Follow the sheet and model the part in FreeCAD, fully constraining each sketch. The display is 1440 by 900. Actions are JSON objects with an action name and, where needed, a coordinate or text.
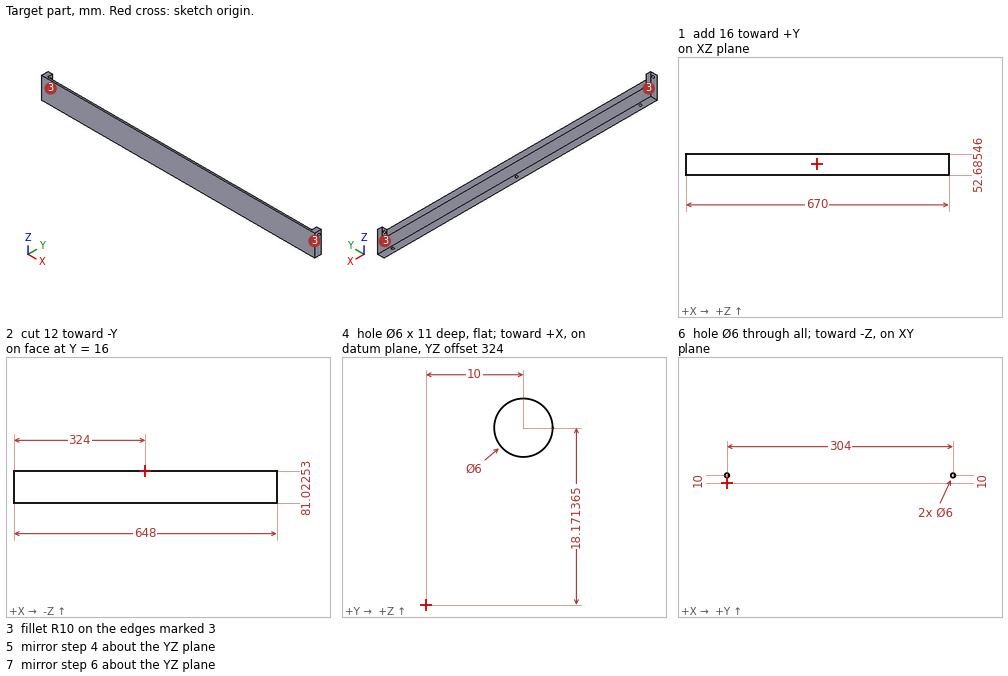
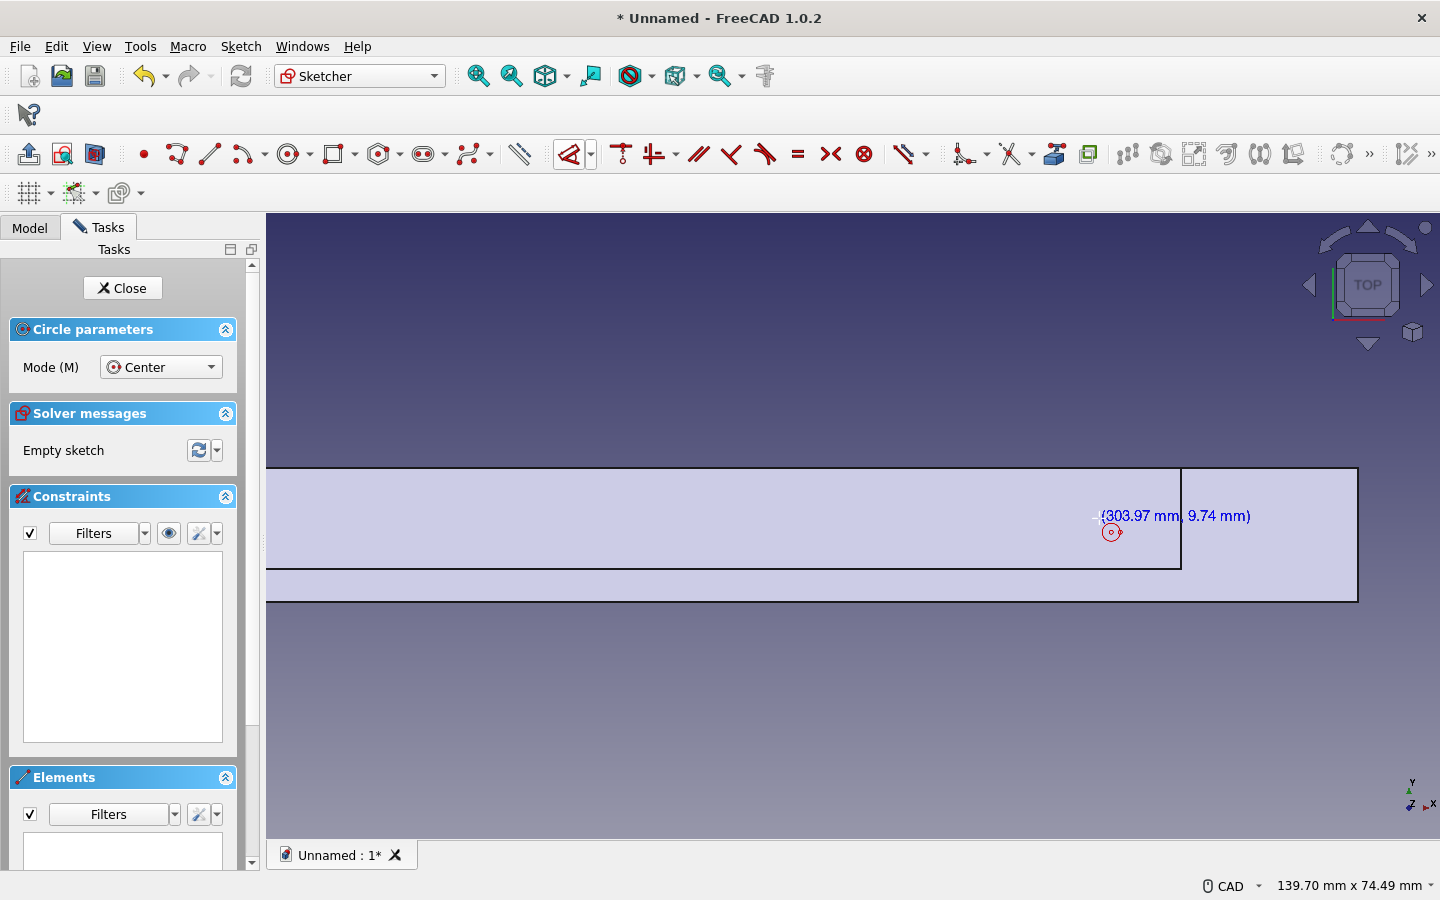
{"action": "scroll", "coordinate": [1100, 519], "scroll_direction": "down", "scroll_amount": 7}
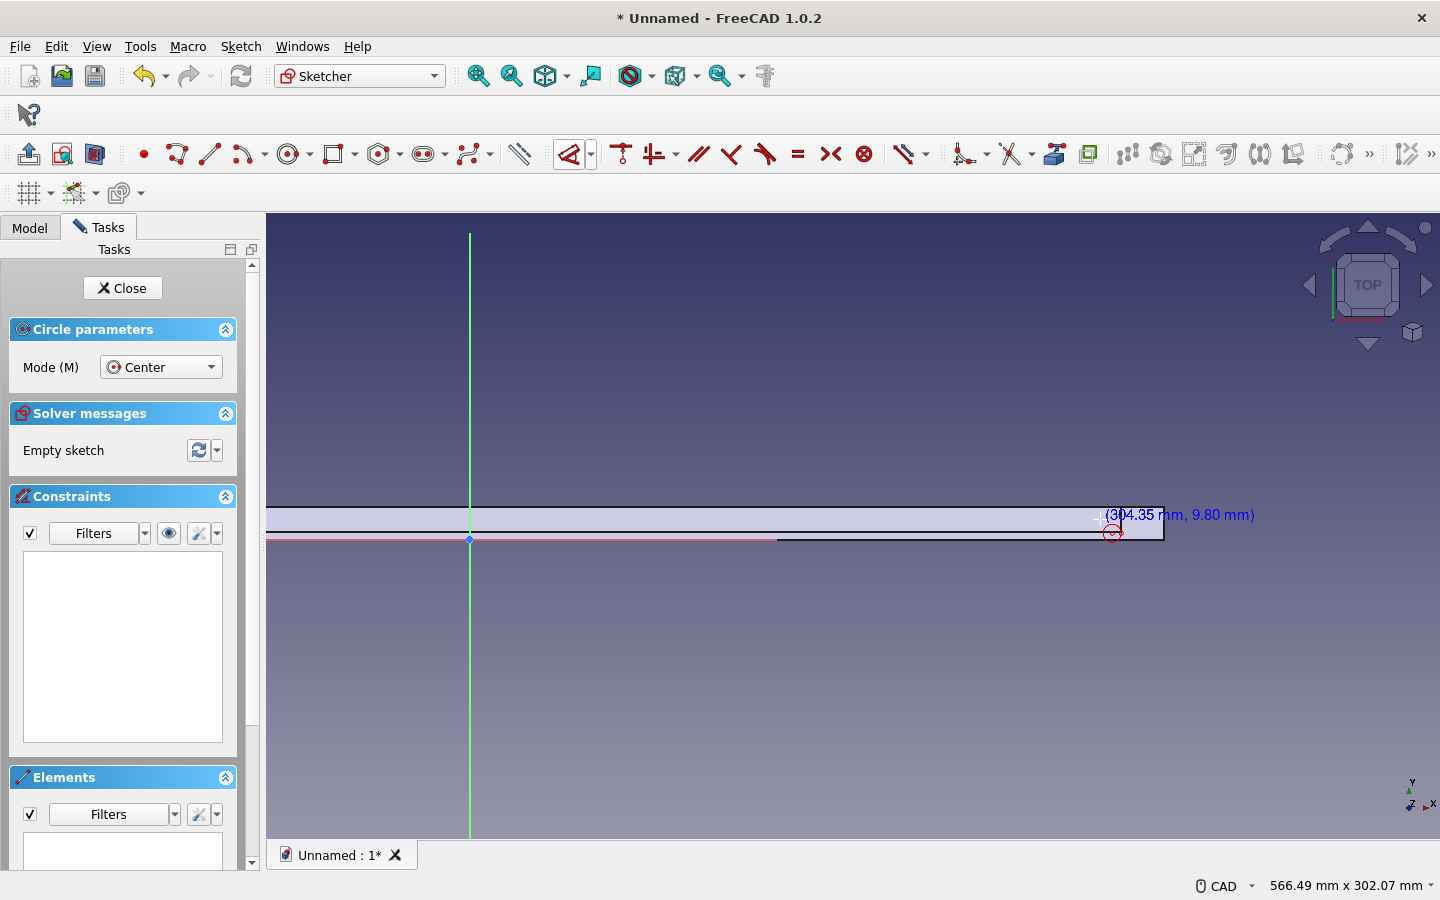
{"action": "left_click", "coordinate": [1100, 519]}
{"action": "mouse_move", "coordinate": [1104, 515]}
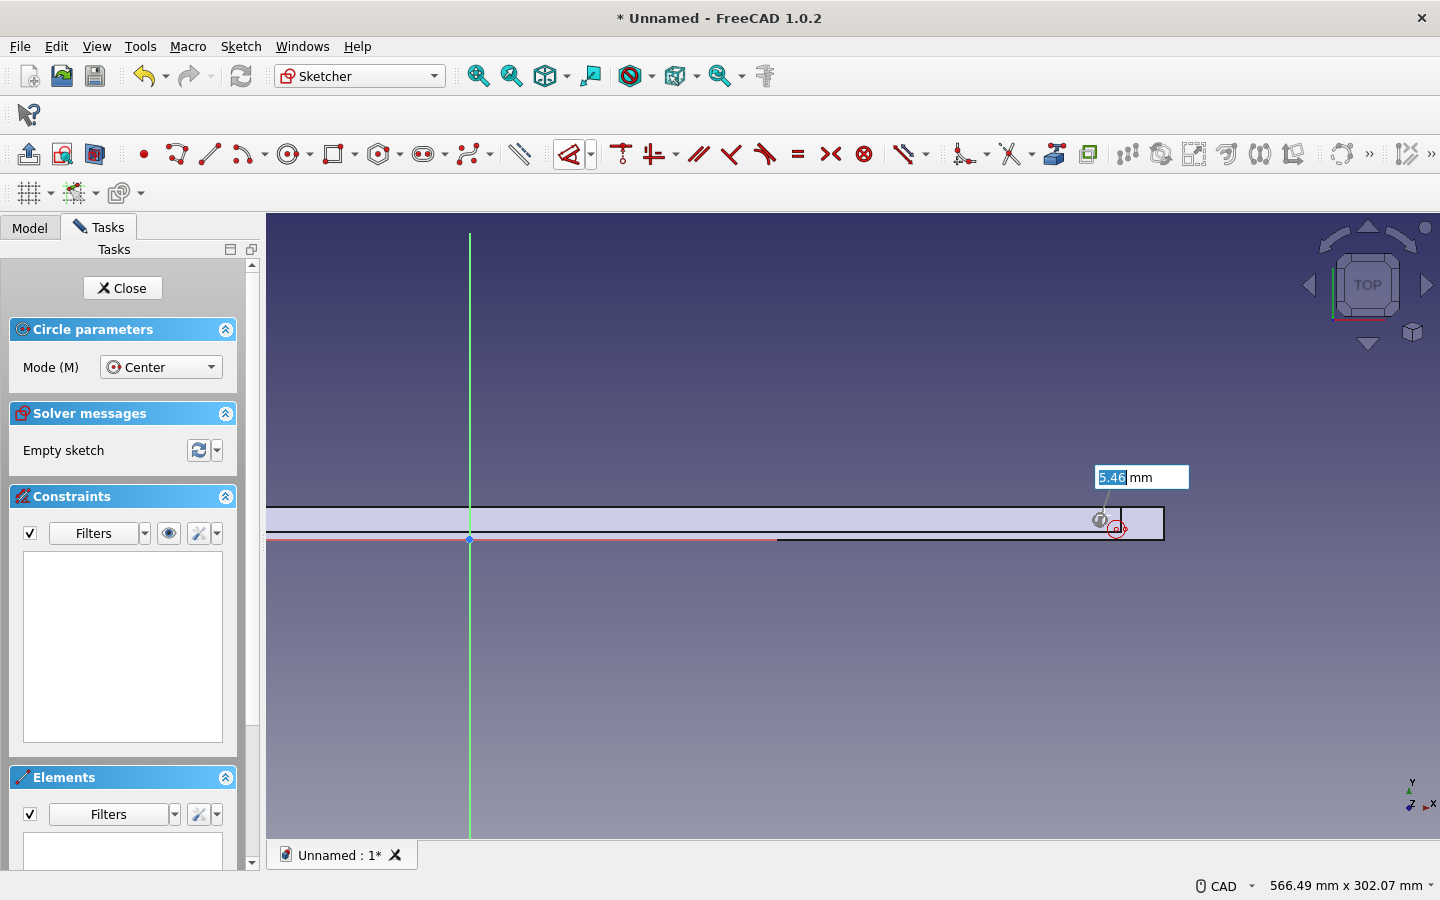
{"action": "type", "text": "6"}
{"action": "key", "text": "Return"}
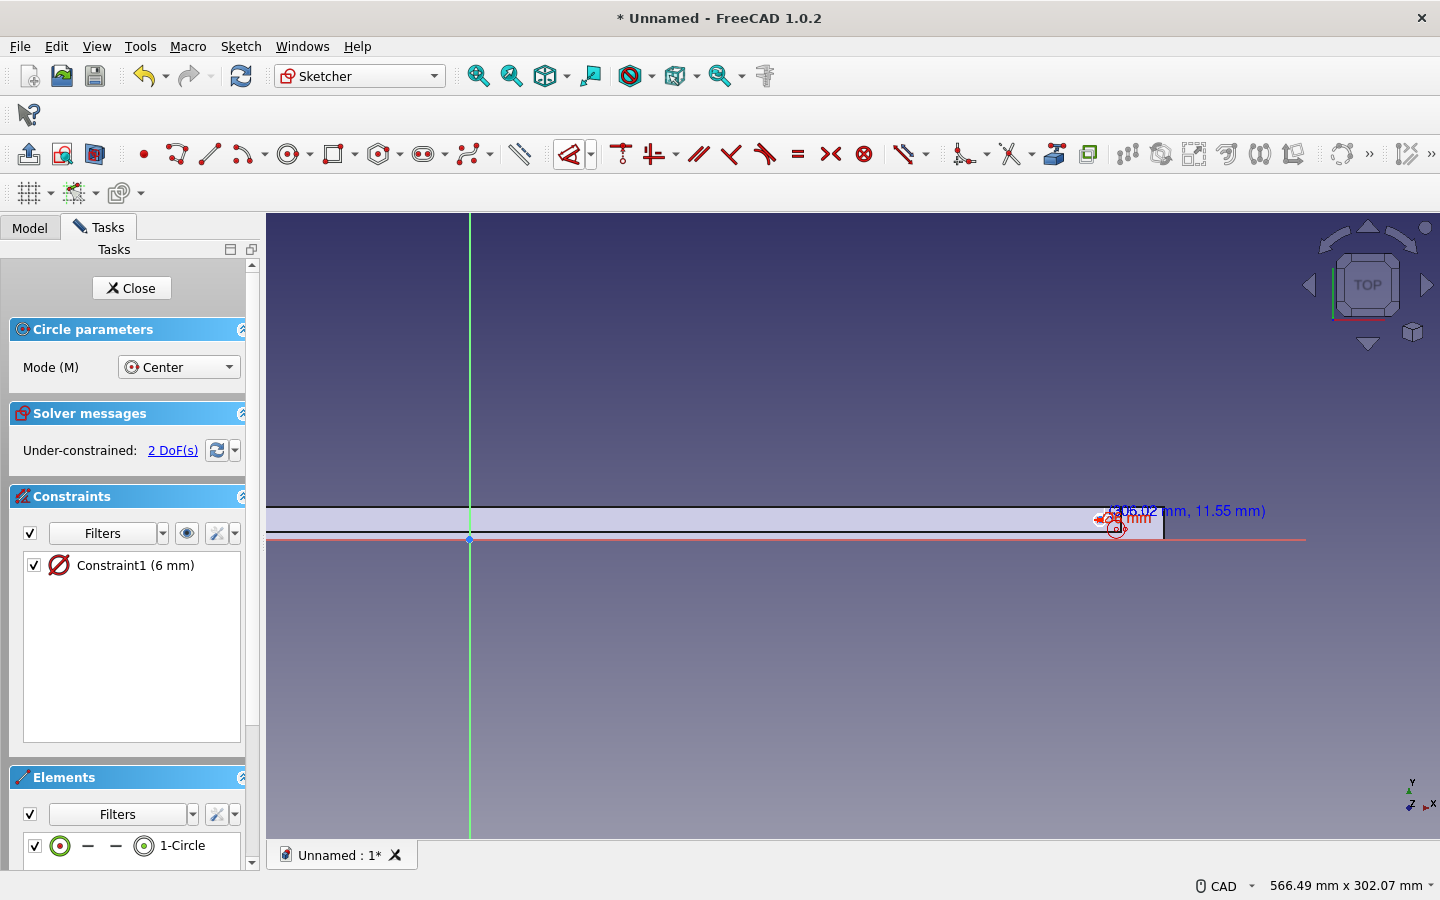
{"action": "scroll", "coordinate": [470, 519], "scroll_direction": "up", "scroll_amount": 7}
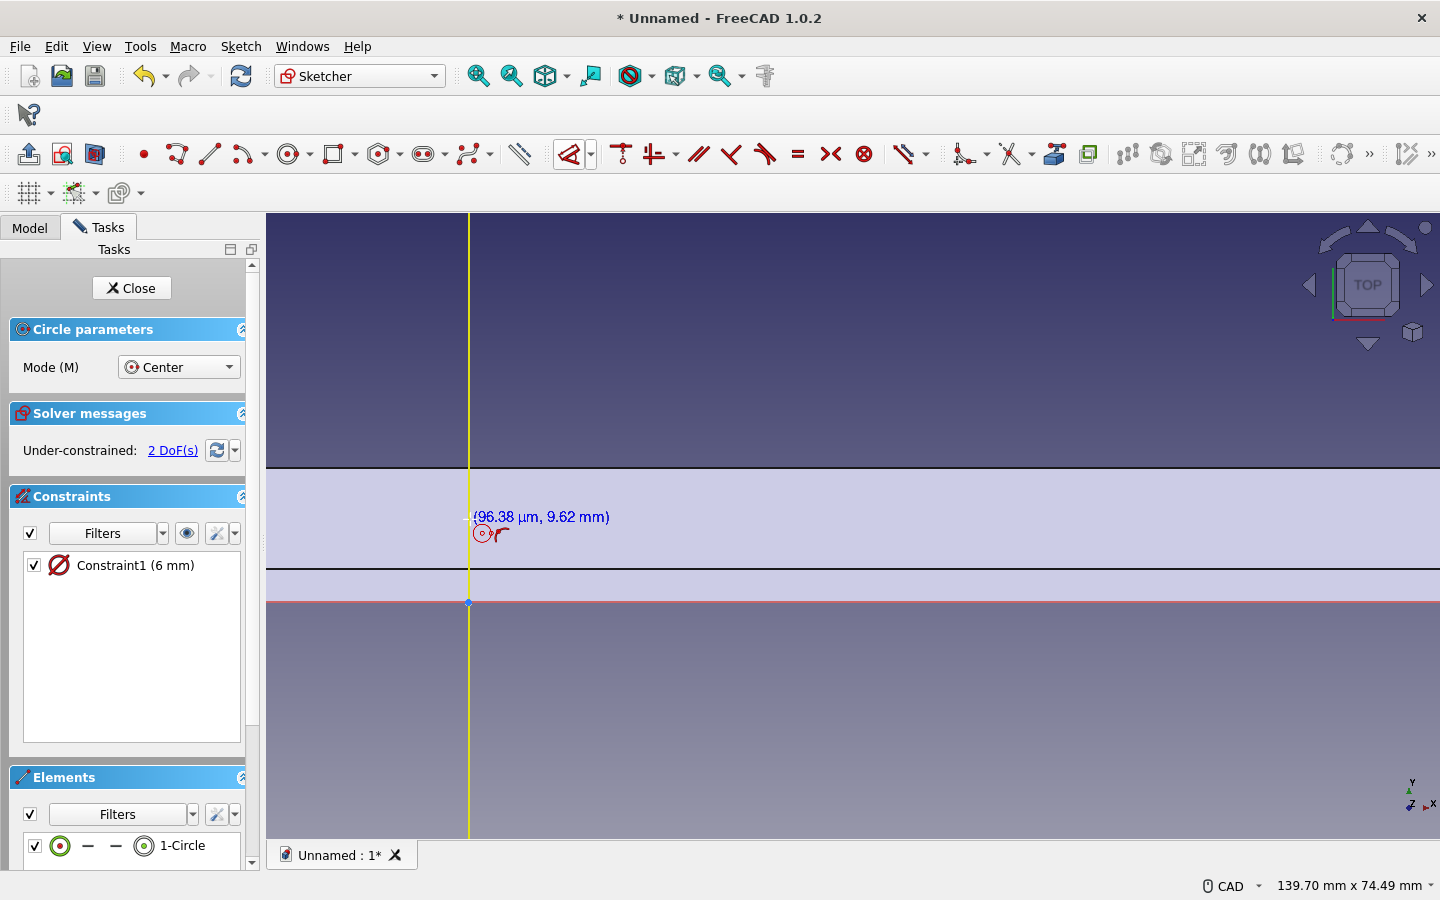
{"action": "scroll", "coordinate": [470, 519], "scroll_direction": "down", "scroll_amount": 7}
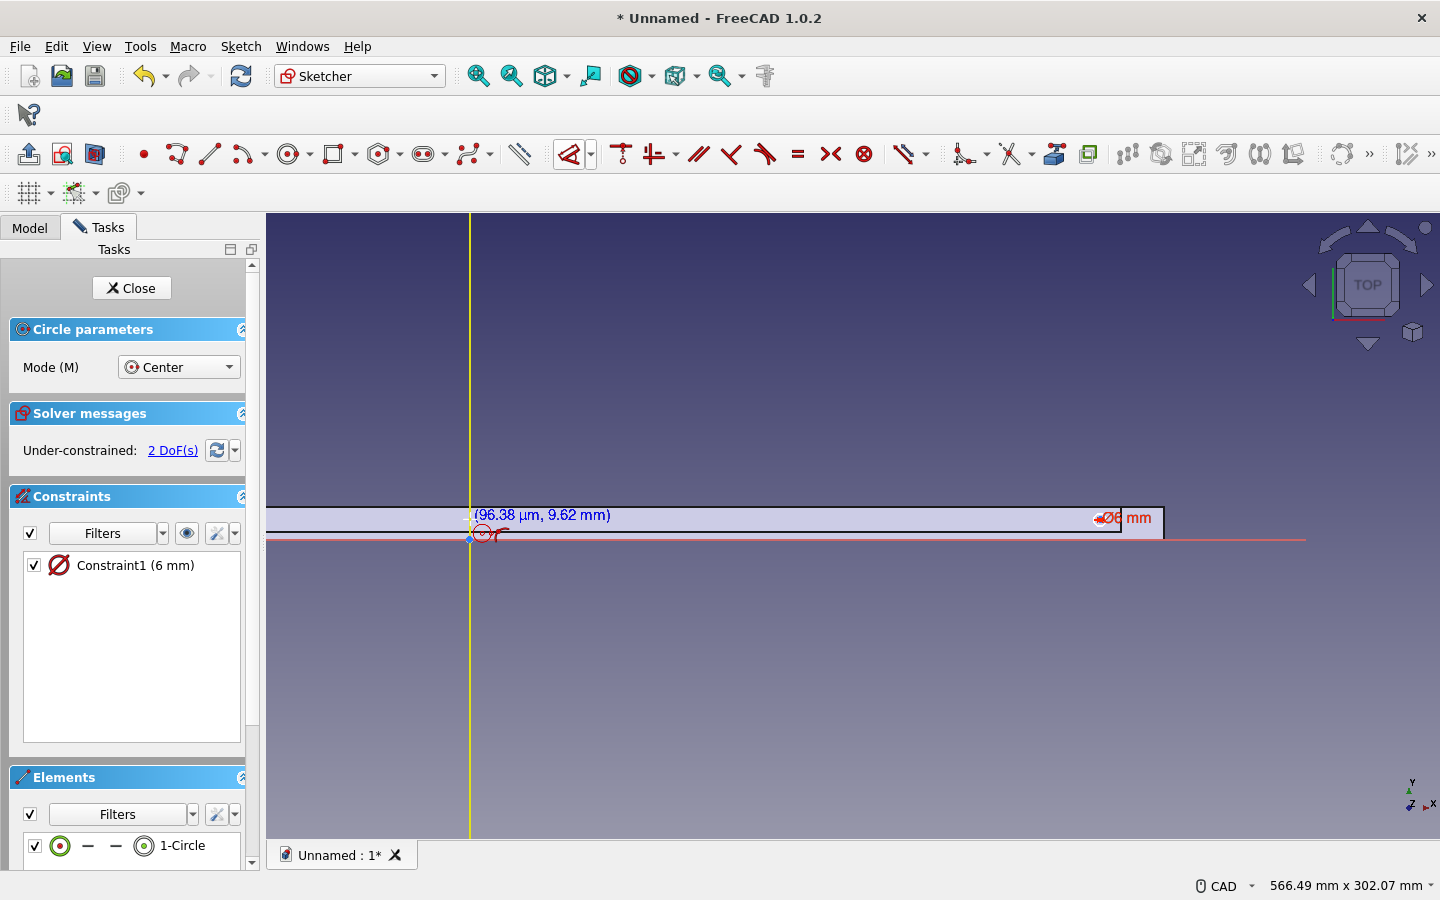
{"action": "left_click", "coordinate": [470, 519]}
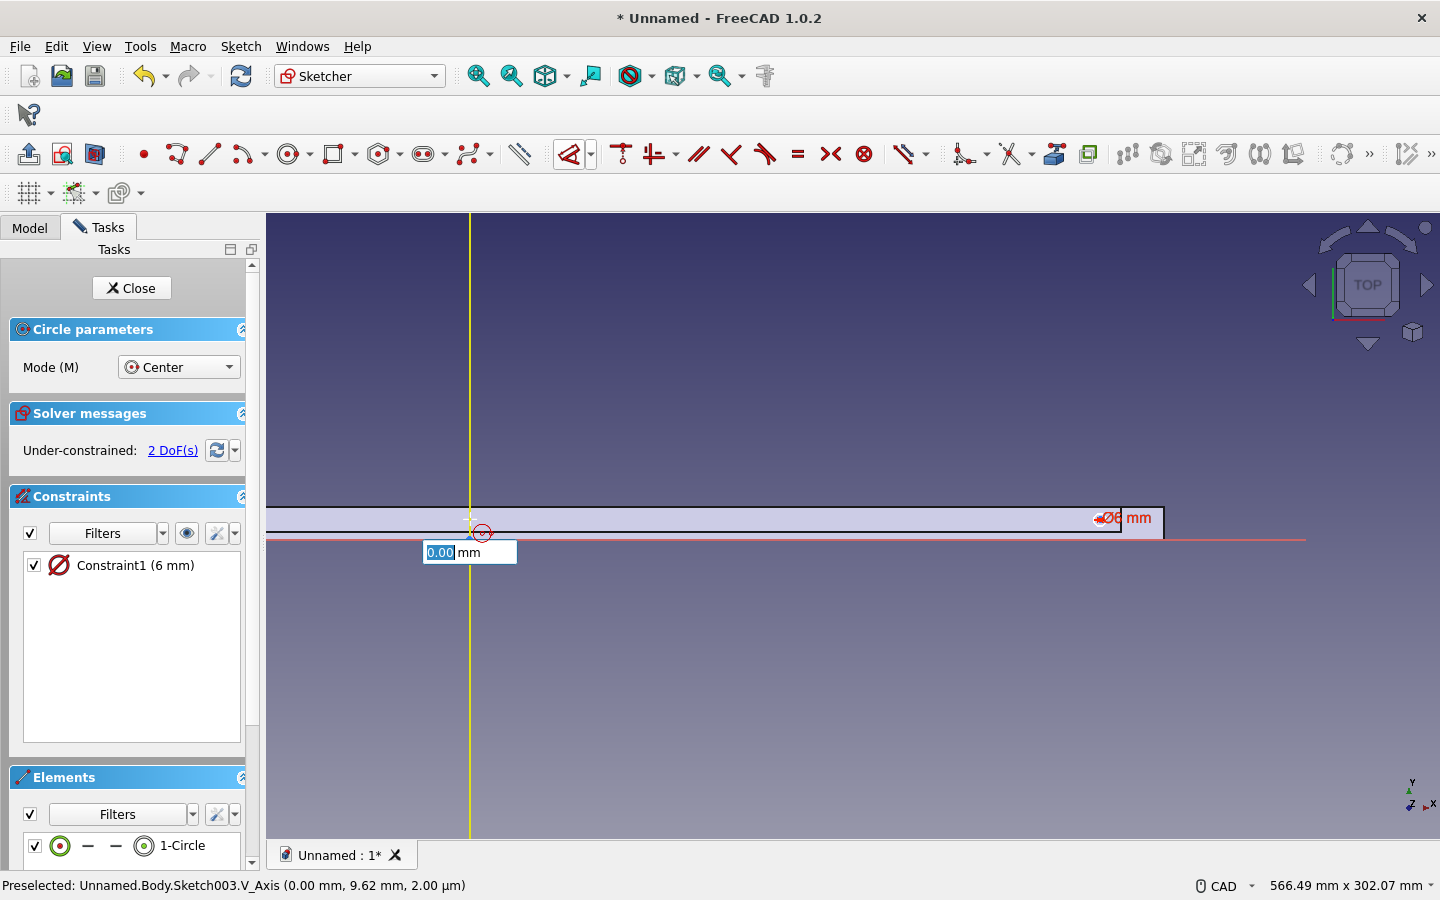
{"action": "scroll", "coordinate": [476, 517], "scroll_direction": "up", "scroll_amount": 5}
{"action": "mouse_move", "coordinate": [475, 516]}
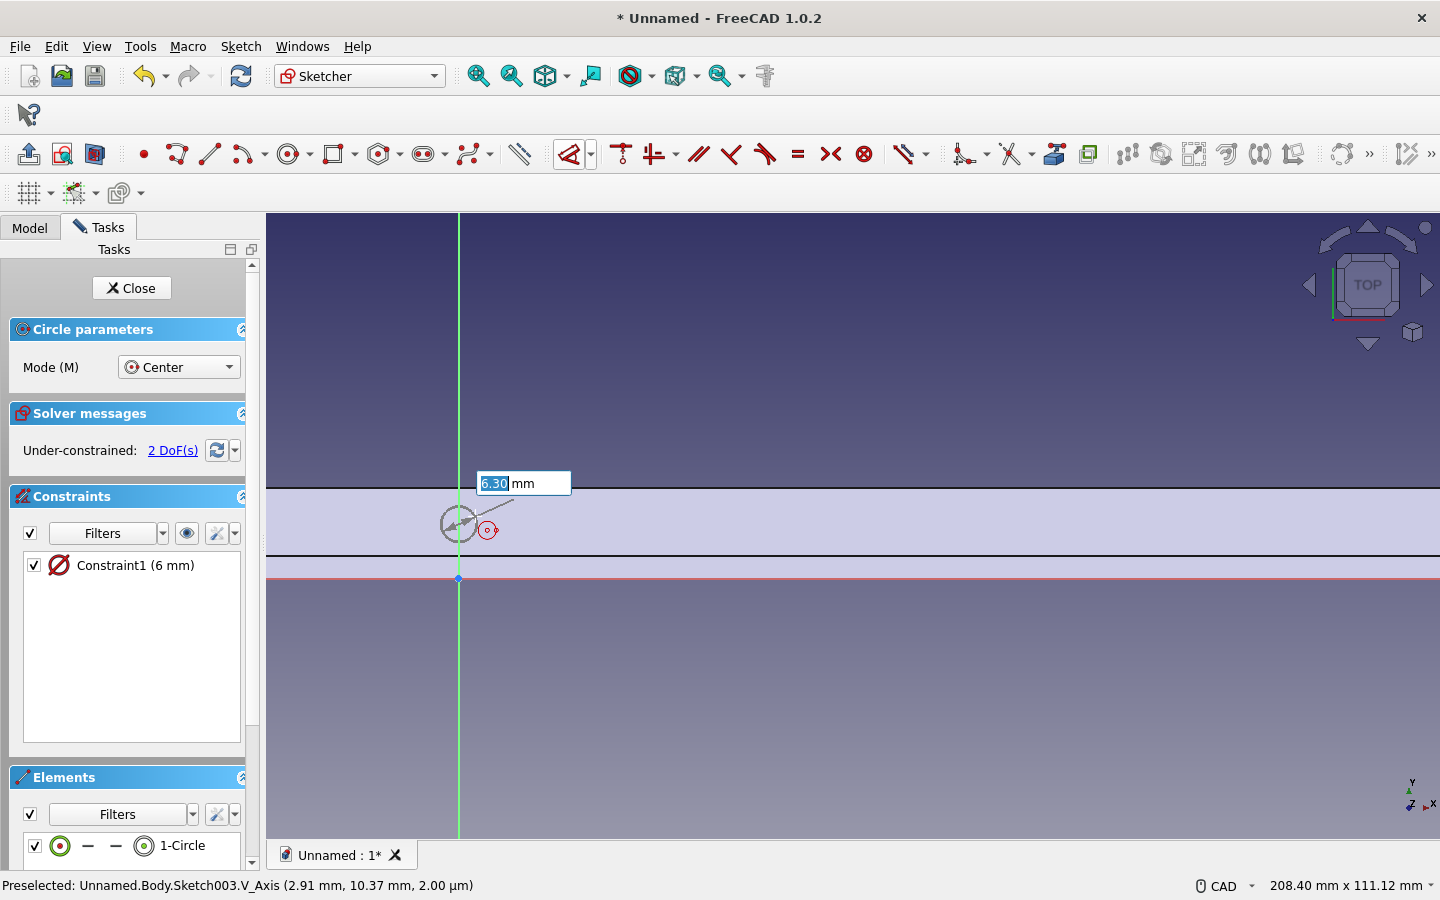
{"action": "type", "text": "6"}
{"action": "key", "text": "Return"}
{"action": "key", "text": "Escape"}